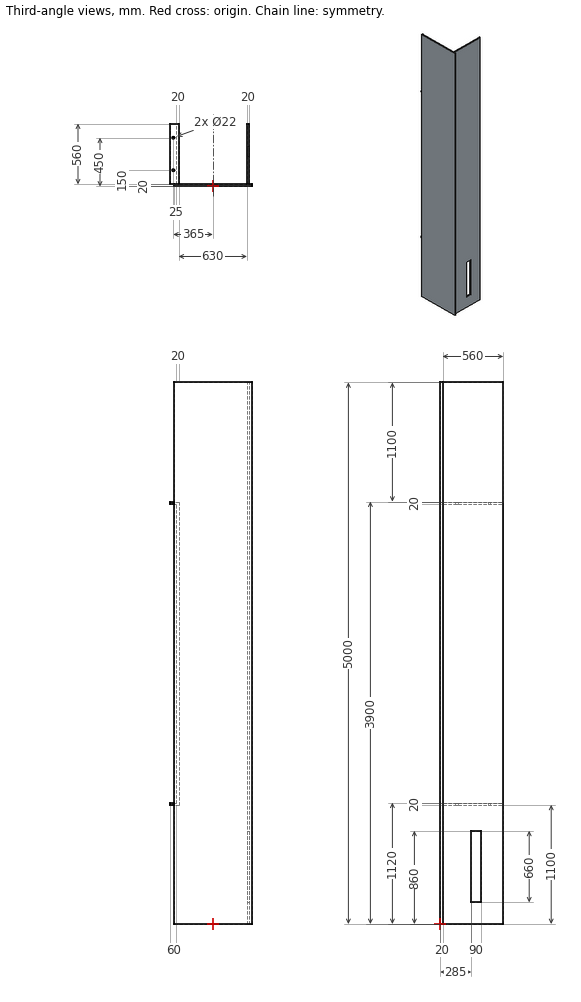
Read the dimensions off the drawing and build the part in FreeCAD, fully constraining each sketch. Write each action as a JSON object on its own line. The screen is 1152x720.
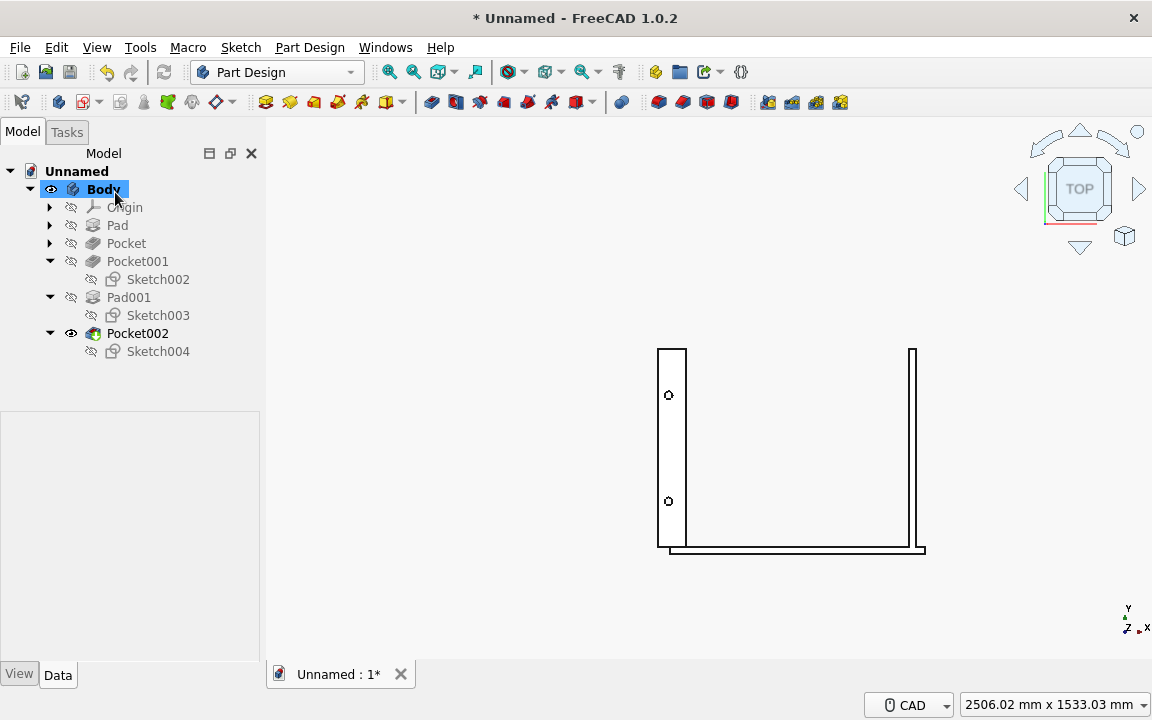
{"action": "key", "text": "0"}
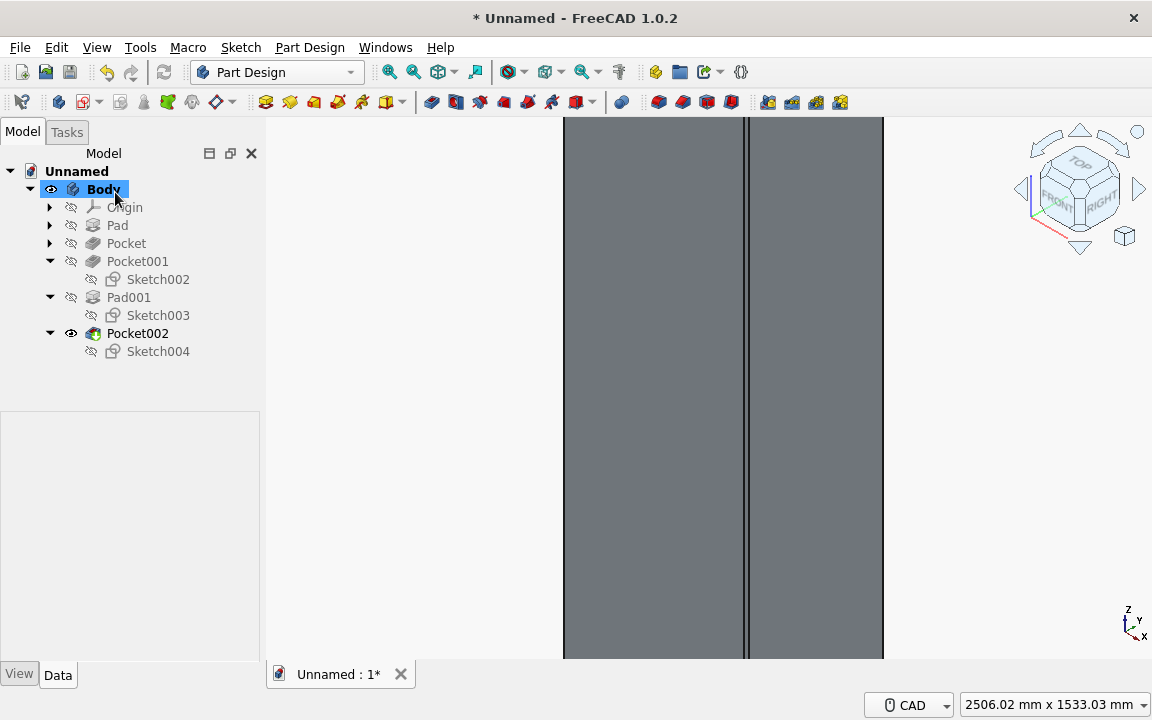
{"action": "left_click", "coordinate": [390, 72]}